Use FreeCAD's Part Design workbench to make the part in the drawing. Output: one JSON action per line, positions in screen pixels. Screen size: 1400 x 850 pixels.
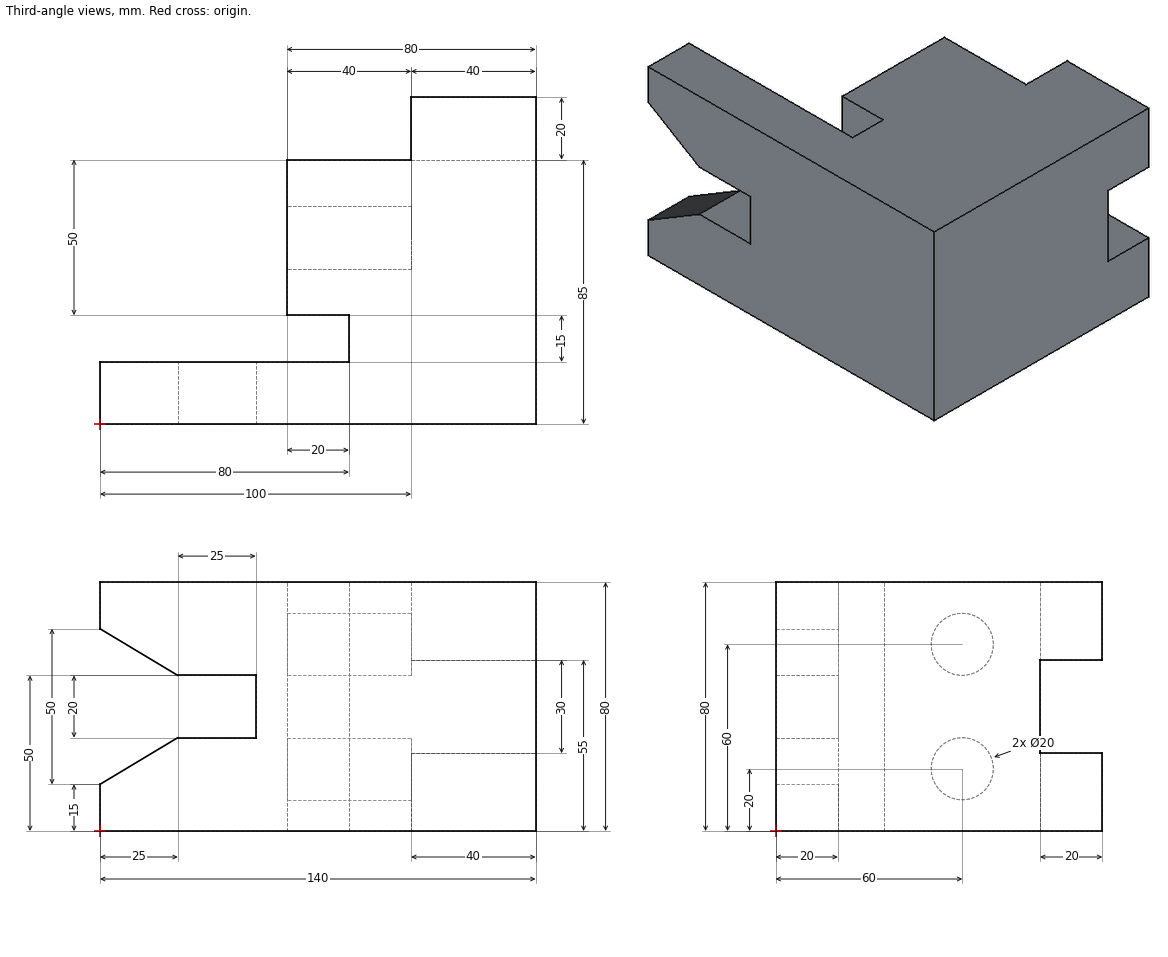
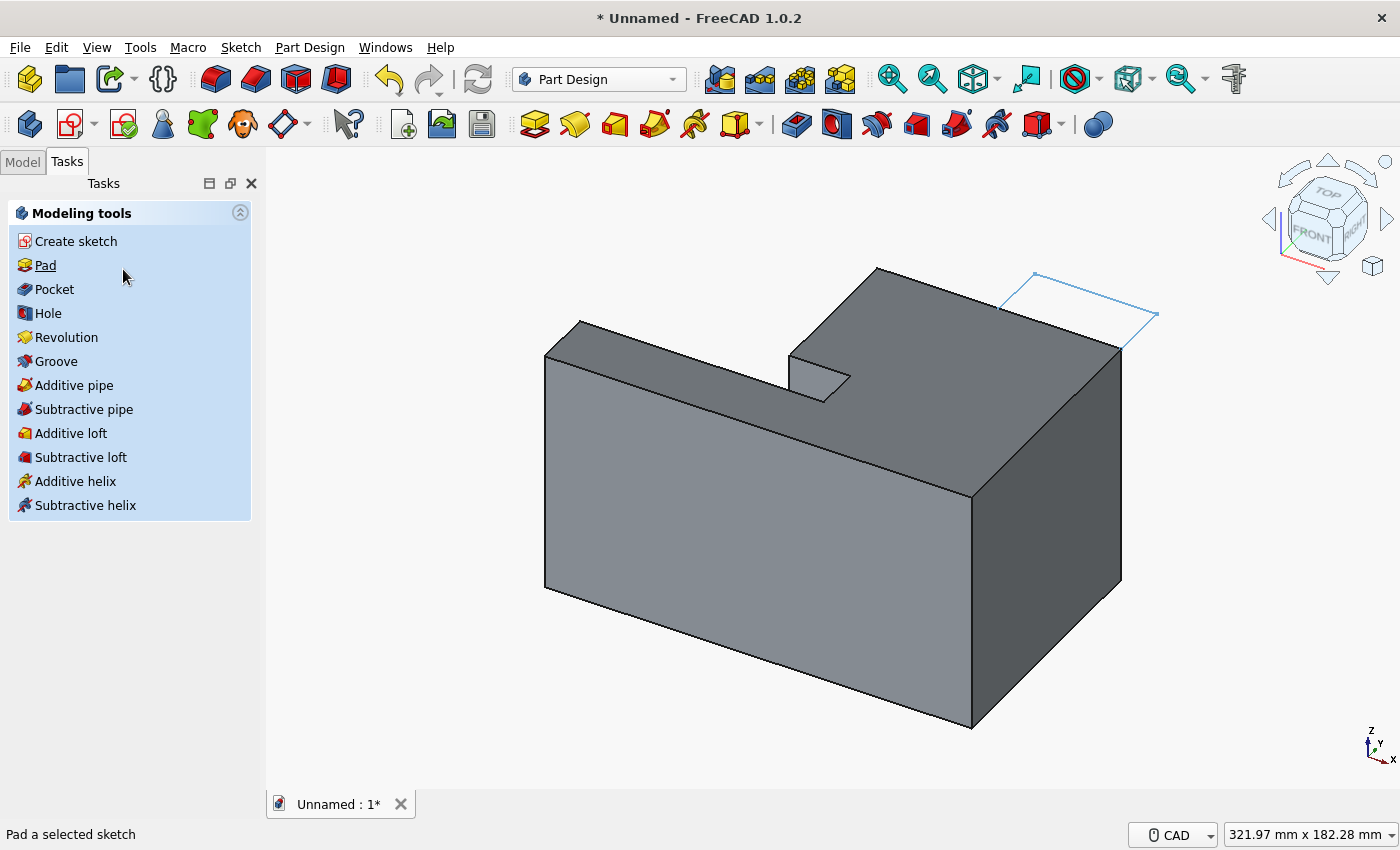
{"action": "left_click", "coordinate": [536, 124]}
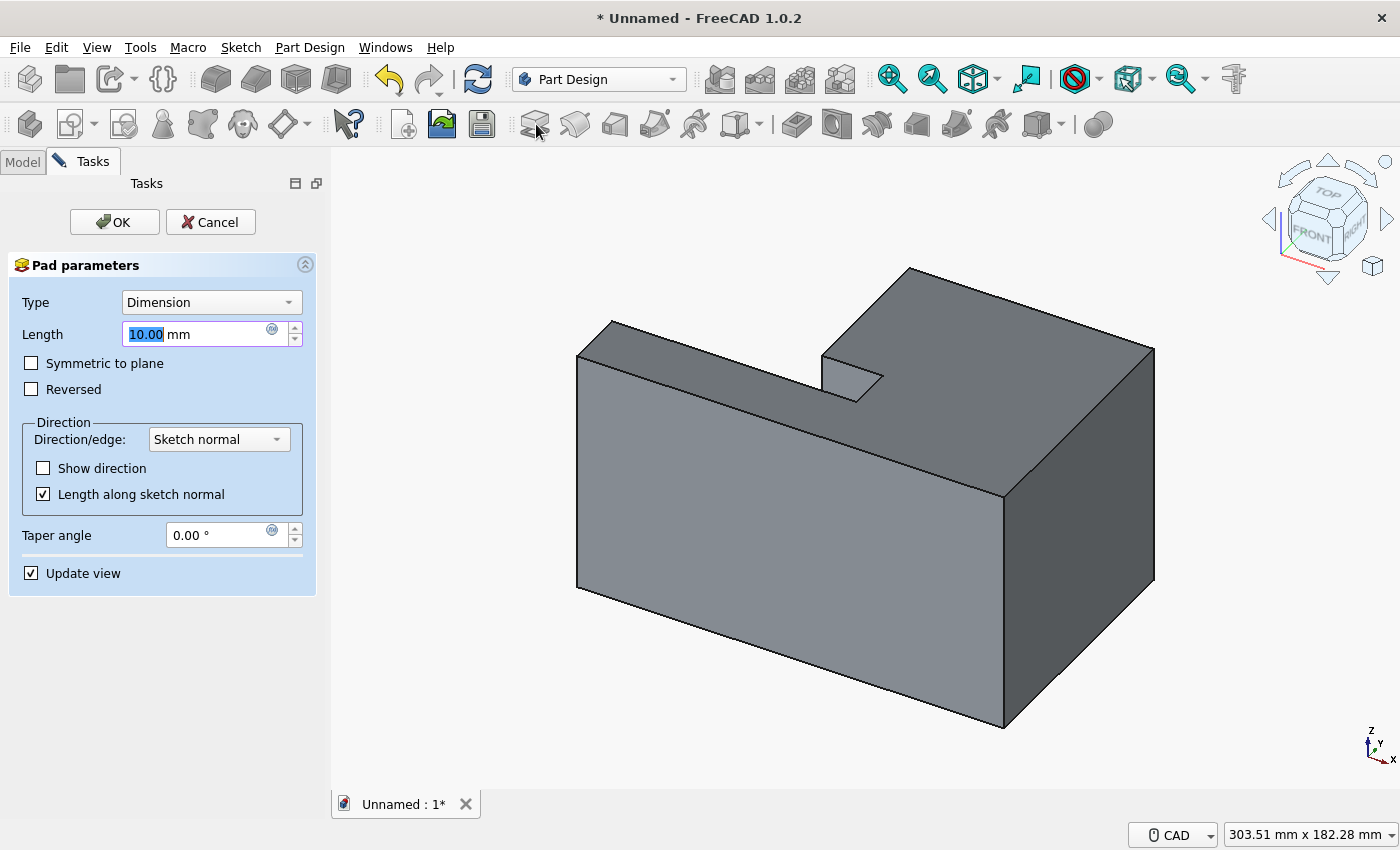
{"action": "type", "text": "80"}
{"action": "key", "text": "Tab"}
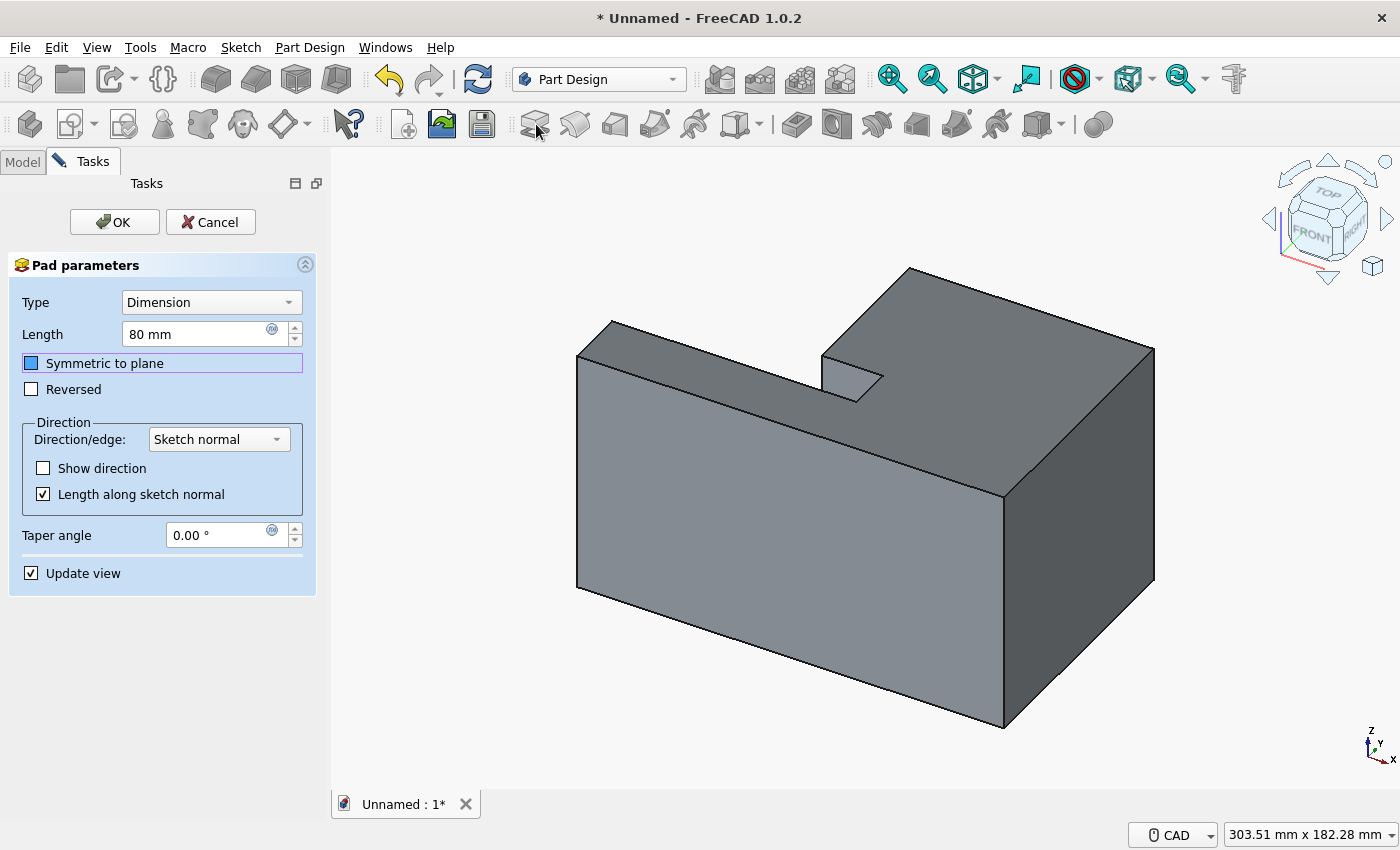
{"action": "left_click", "coordinate": [30, 389]}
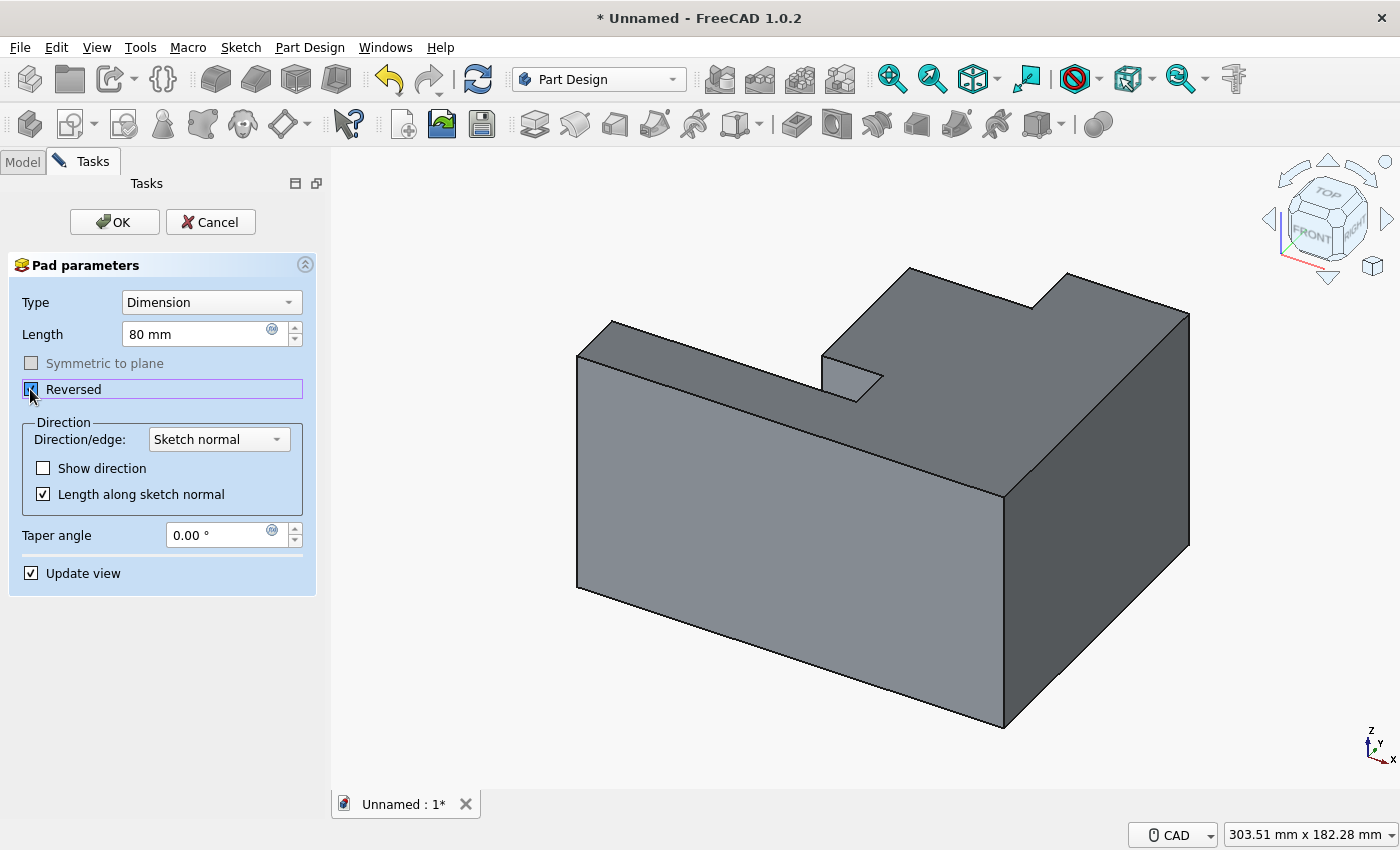
{"action": "left_click", "coordinate": [115, 222]}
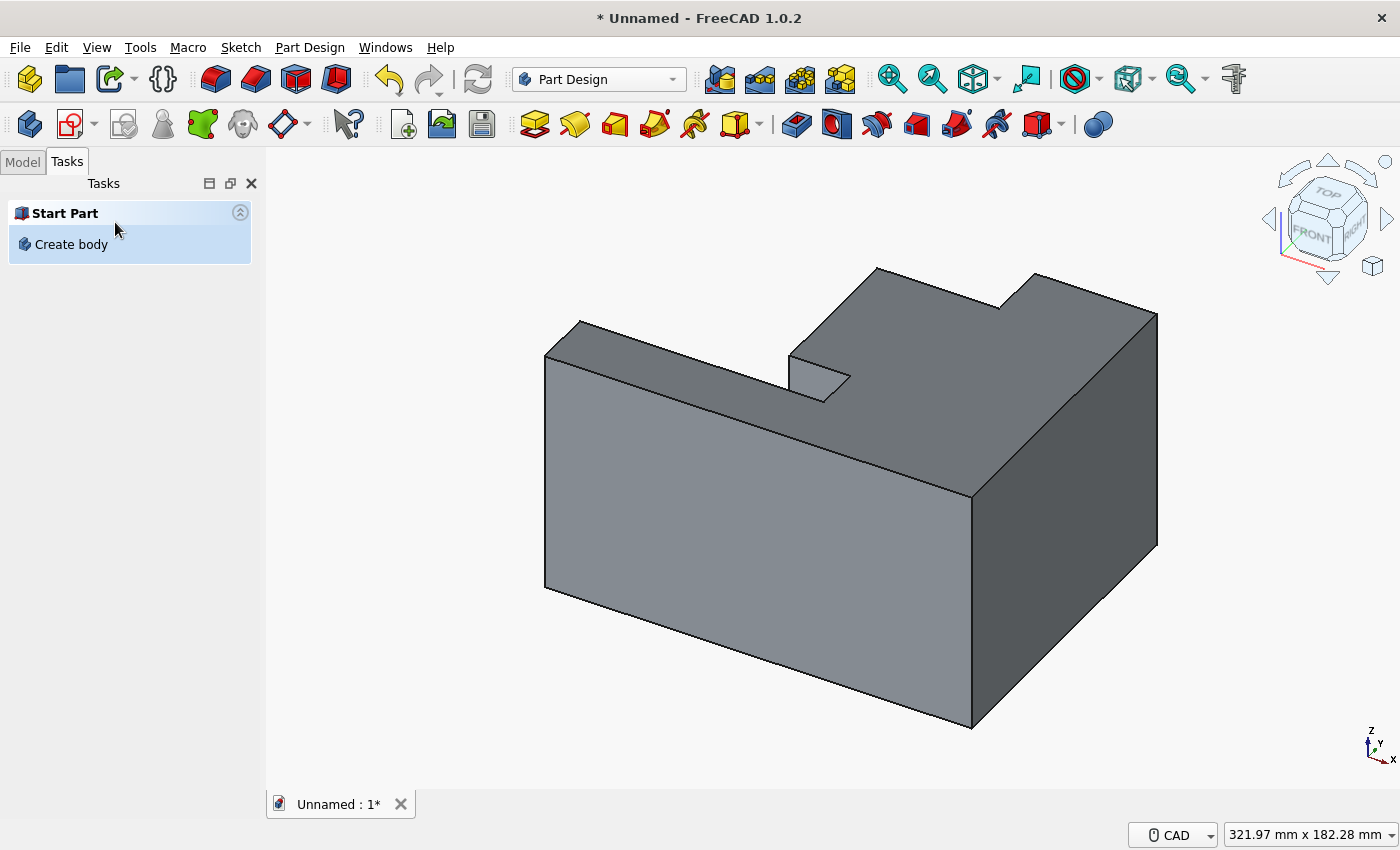
{"action": "key", "text": "4"}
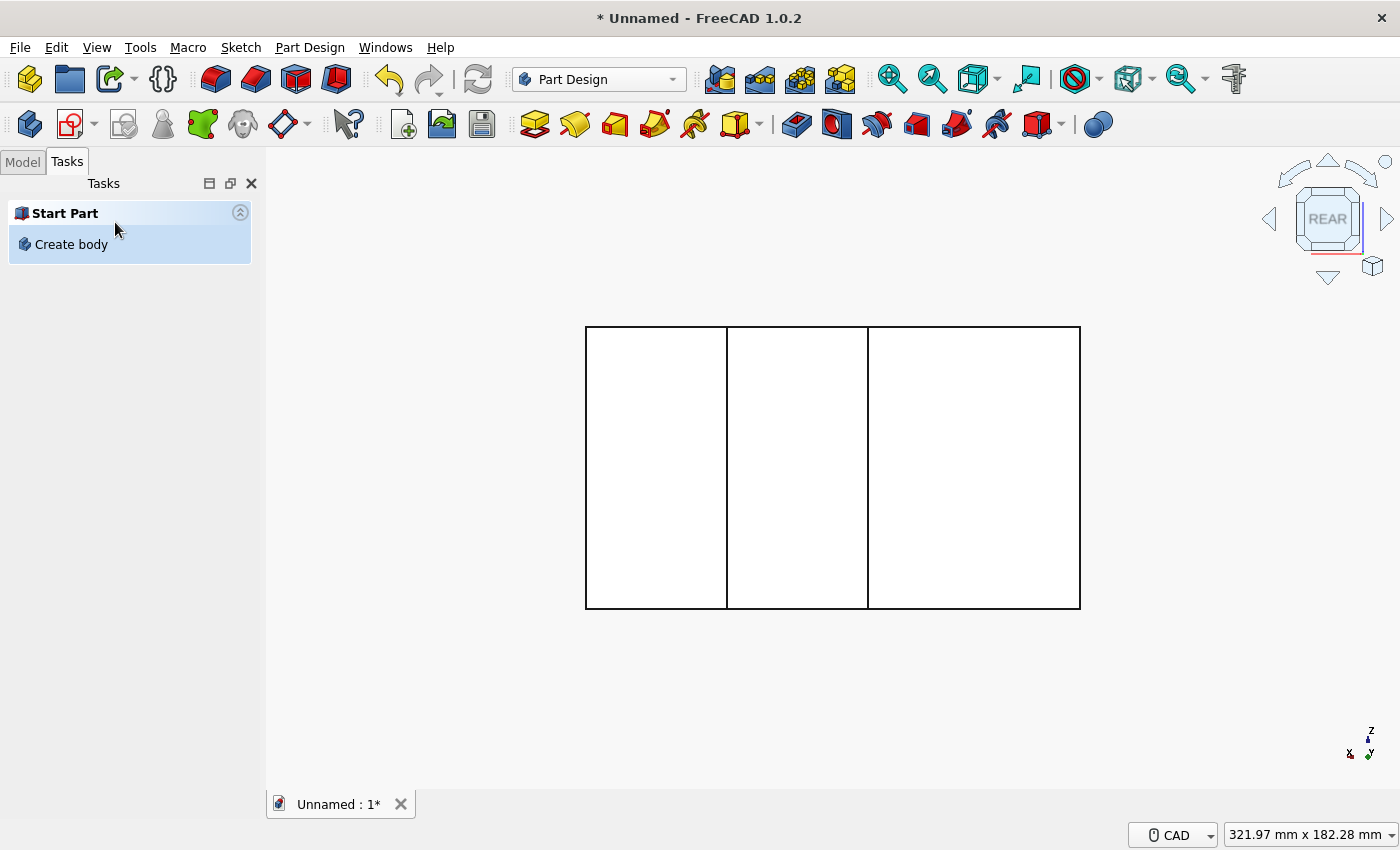
{"action": "key", "text": "v f"}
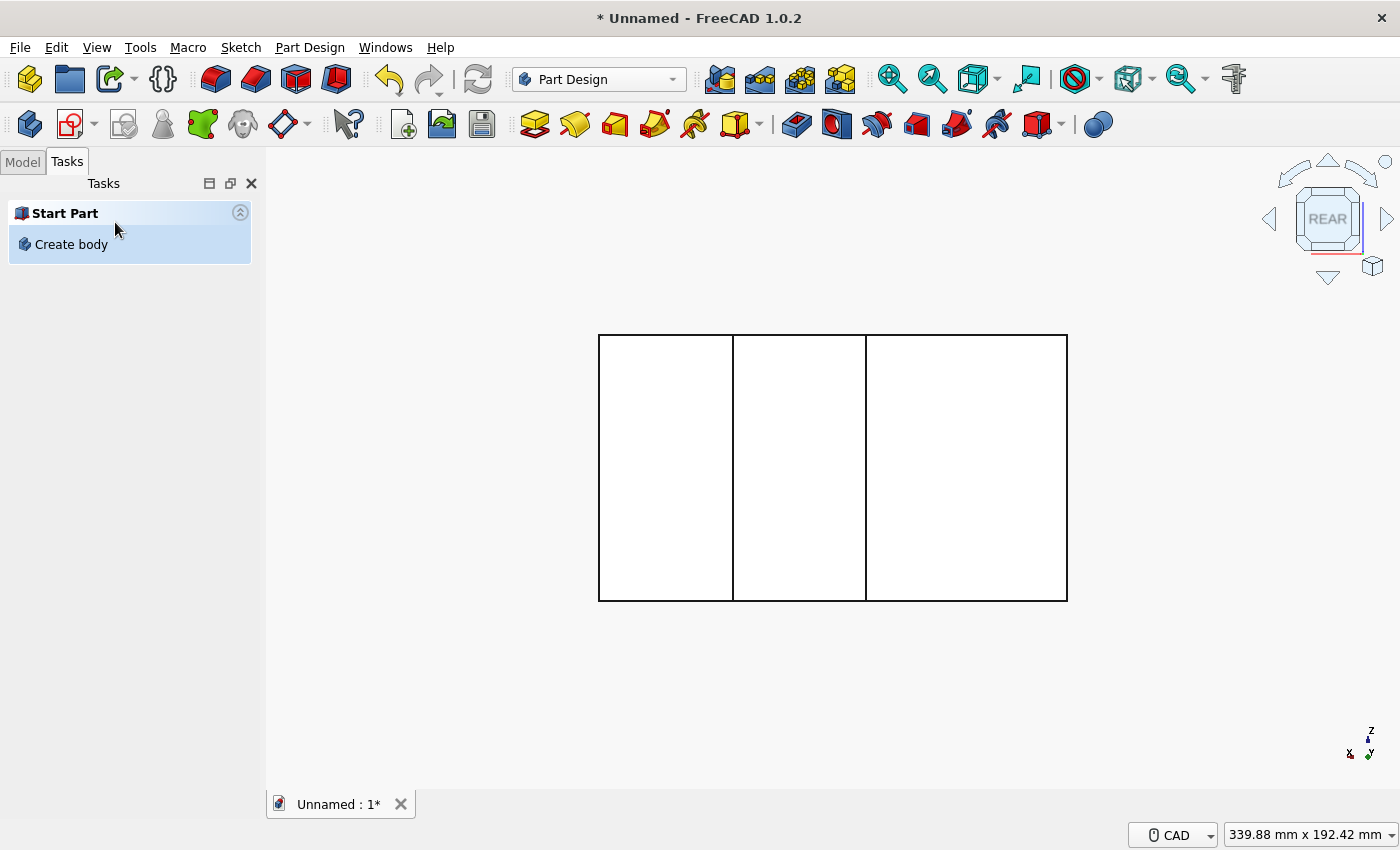
{"action": "left_click", "coordinate": [666, 429]}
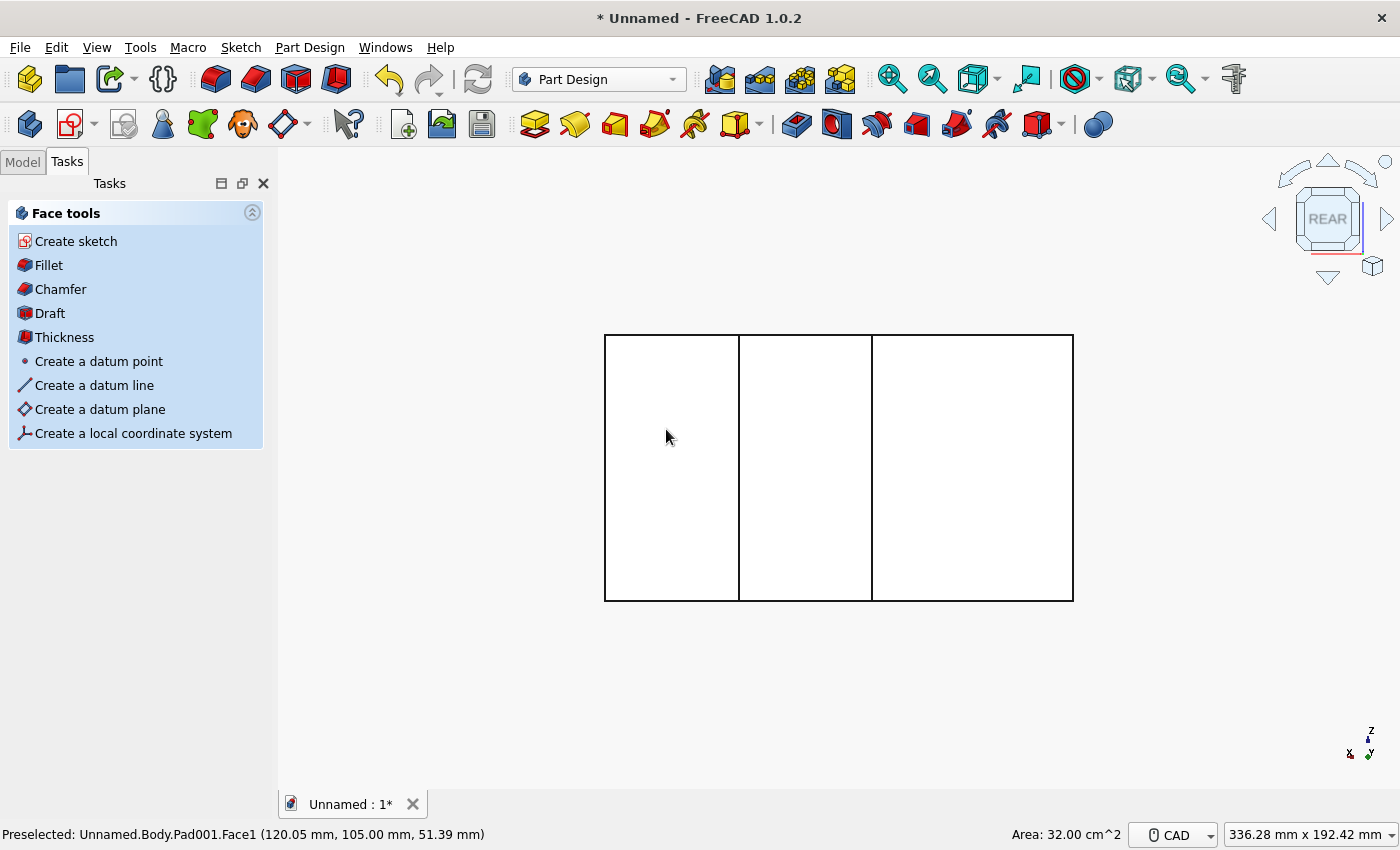
{"action": "left_click", "coordinate": [70, 124]}